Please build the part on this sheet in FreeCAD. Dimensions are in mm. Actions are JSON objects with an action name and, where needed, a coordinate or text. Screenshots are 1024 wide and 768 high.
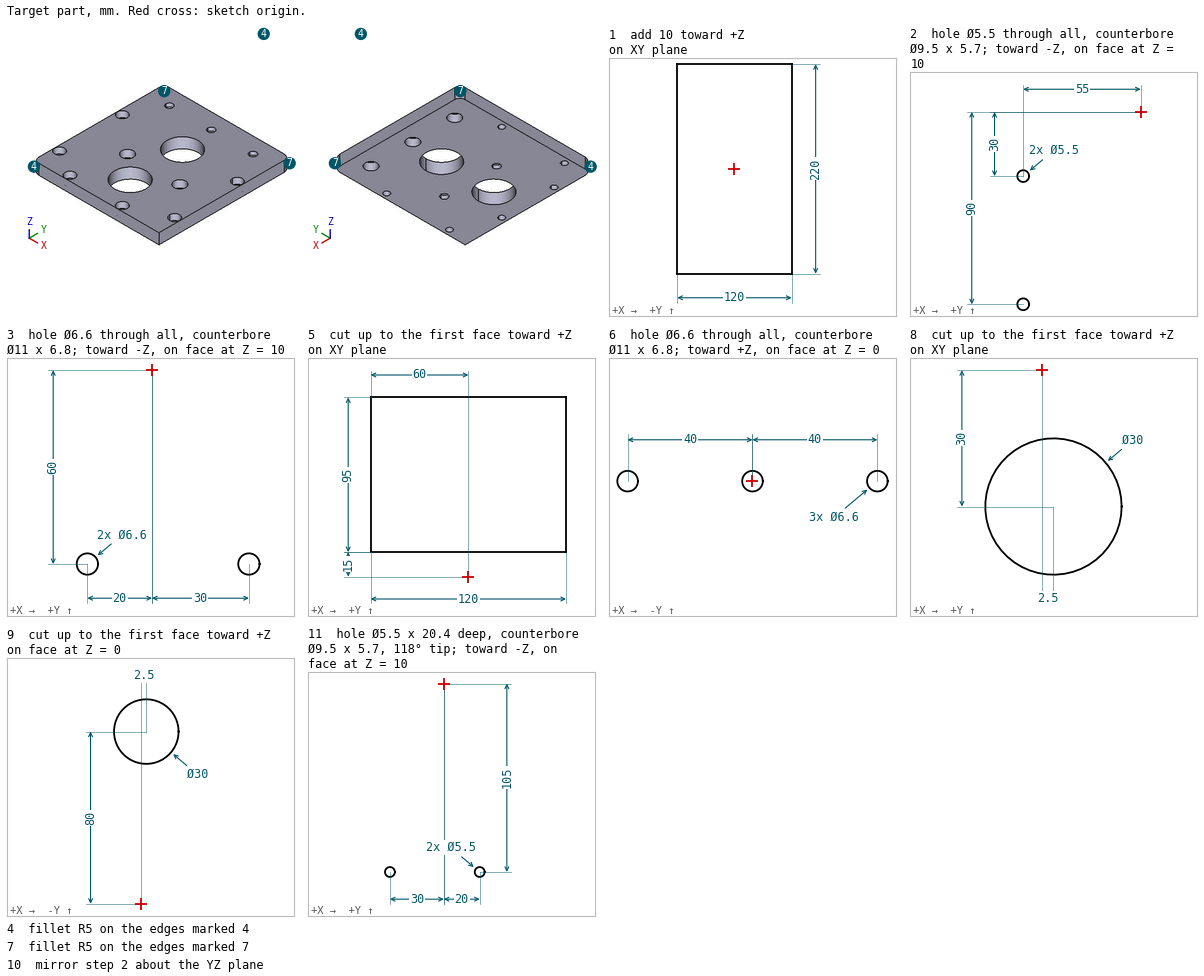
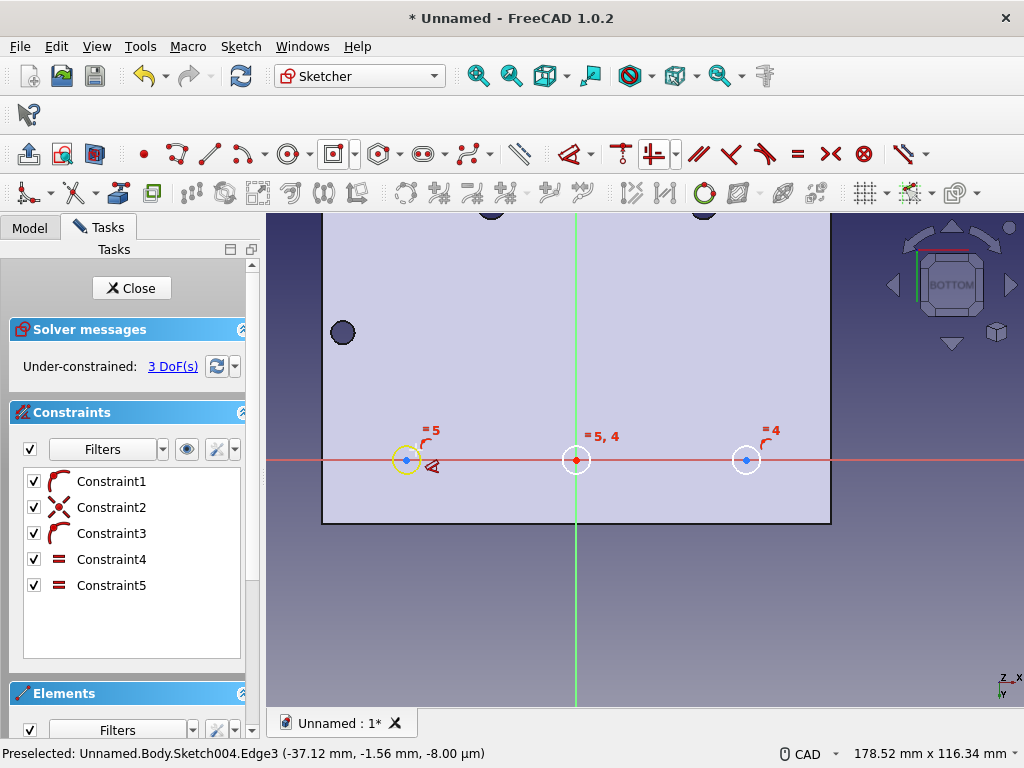
{"action": "scroll", "coordinate": [756, 450], "scroll_direction": "up", "scroll_amount": 2}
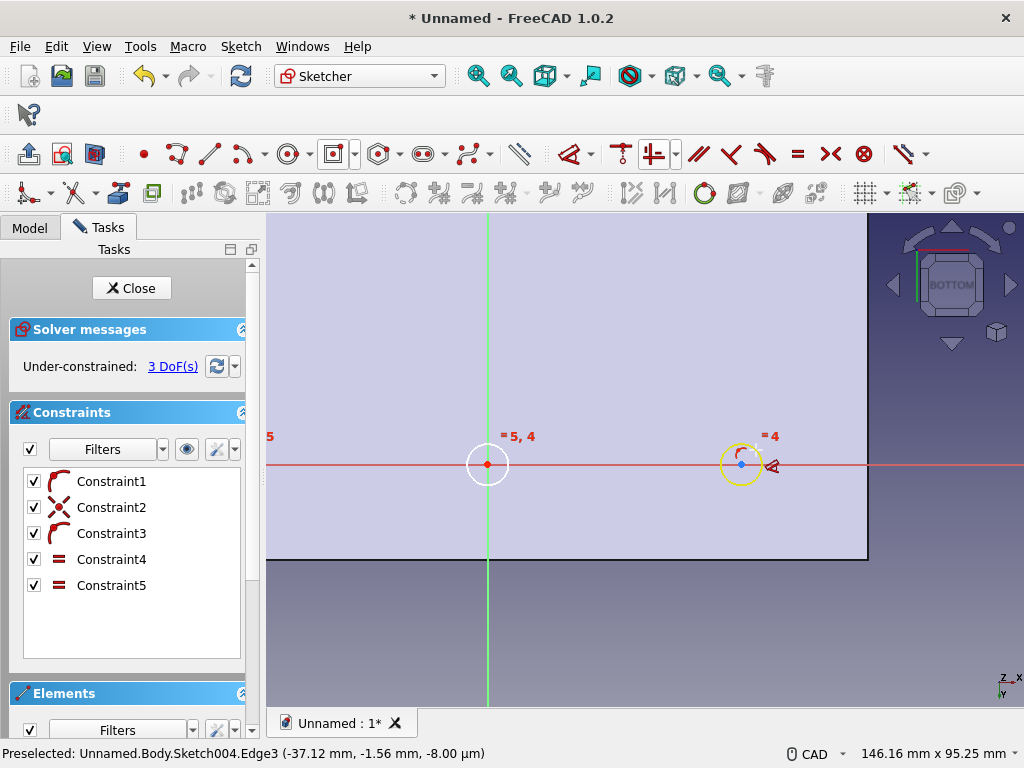
{"action": "left_click", "coordinate": [756, 450]}
{"action": "left_click", "coordinate": [779, 427]}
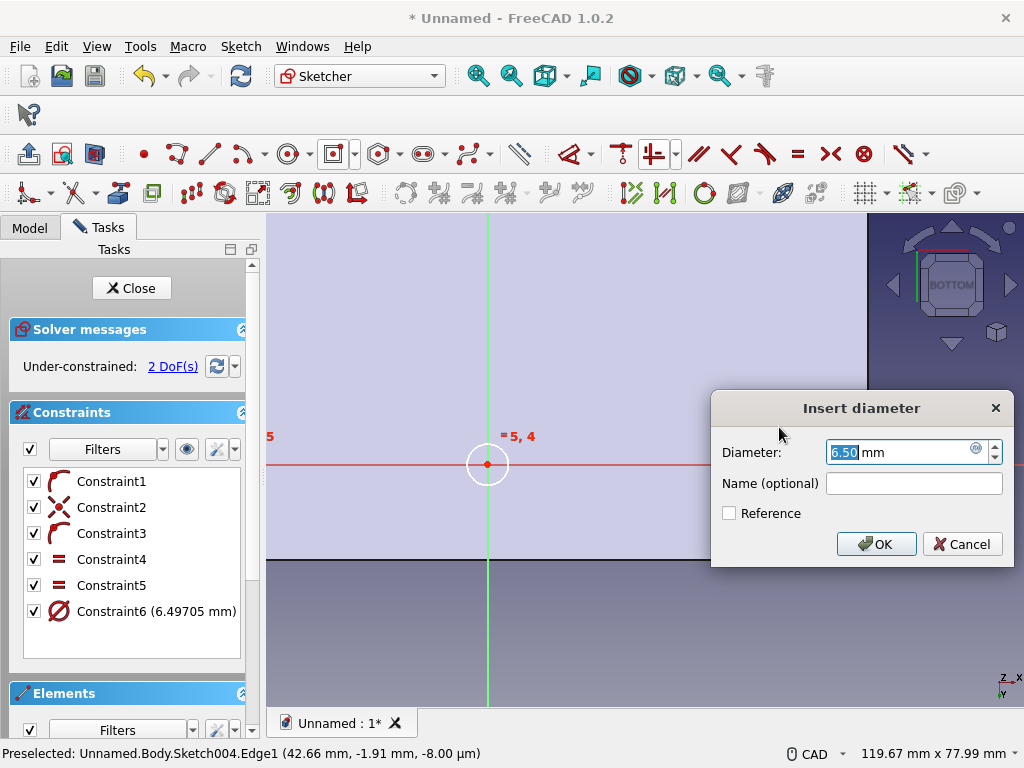
{"action": "type", "text": "6.6"}
{"action": "key", "text": "Return"}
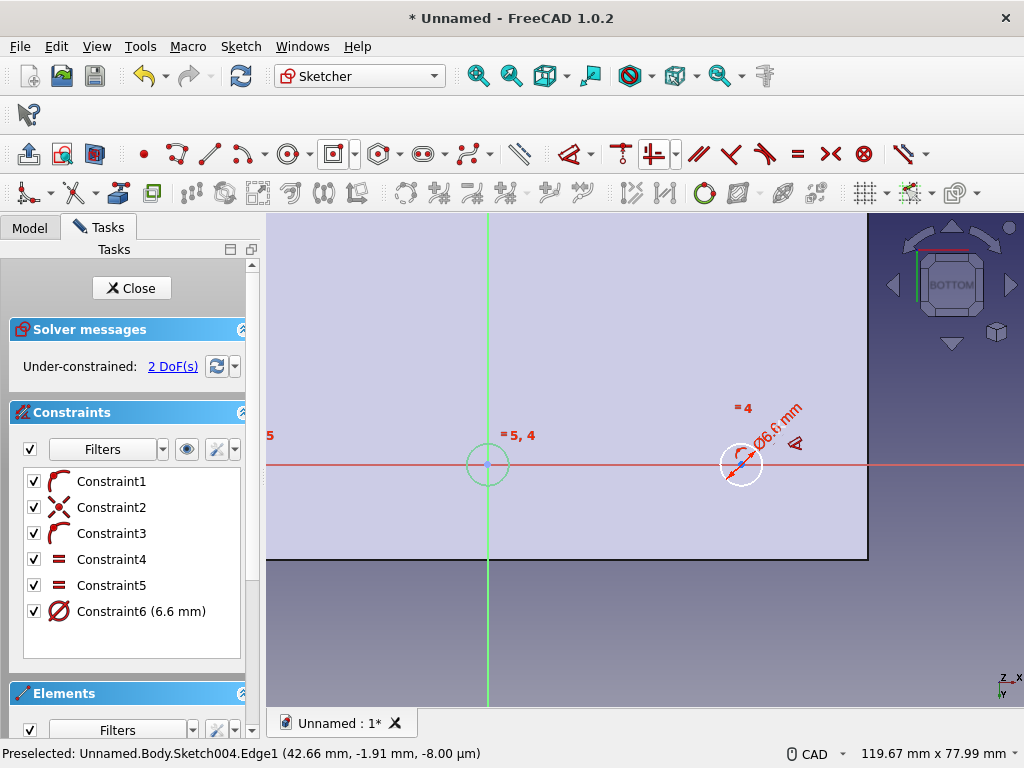
{"action": "left_click", "coordinate": [741, 465]}
{"action": "left_click", "coordinate": [615, 499]}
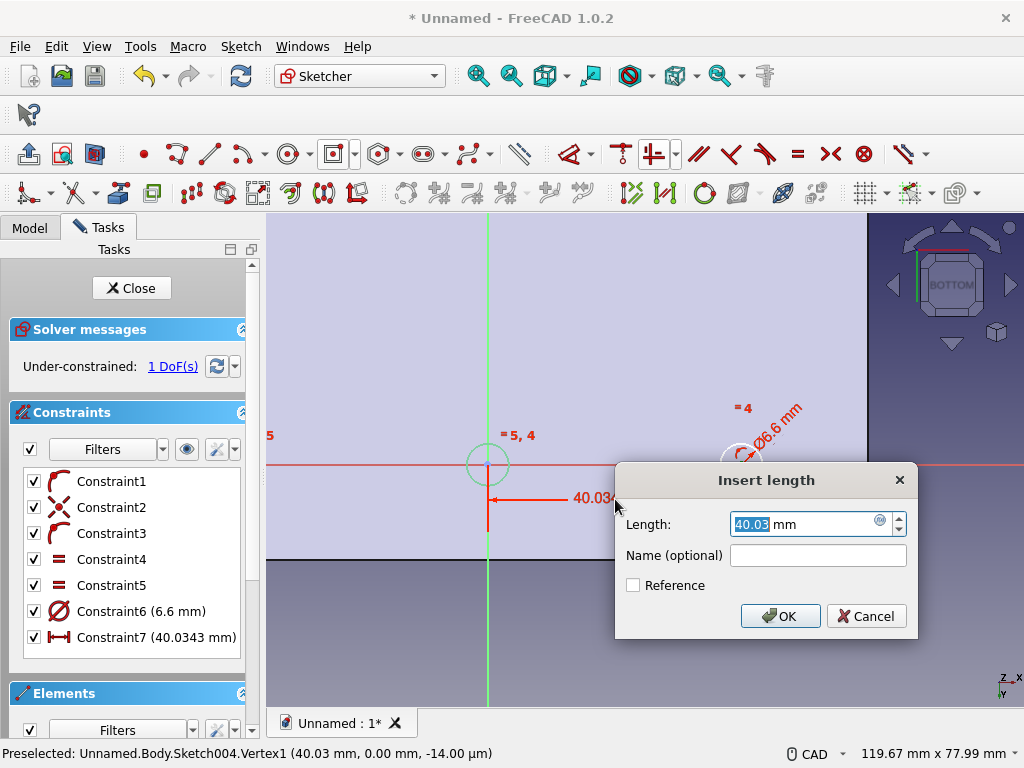
{"action": "type", "text": "40"}
{"action": "key", "text": "Return"}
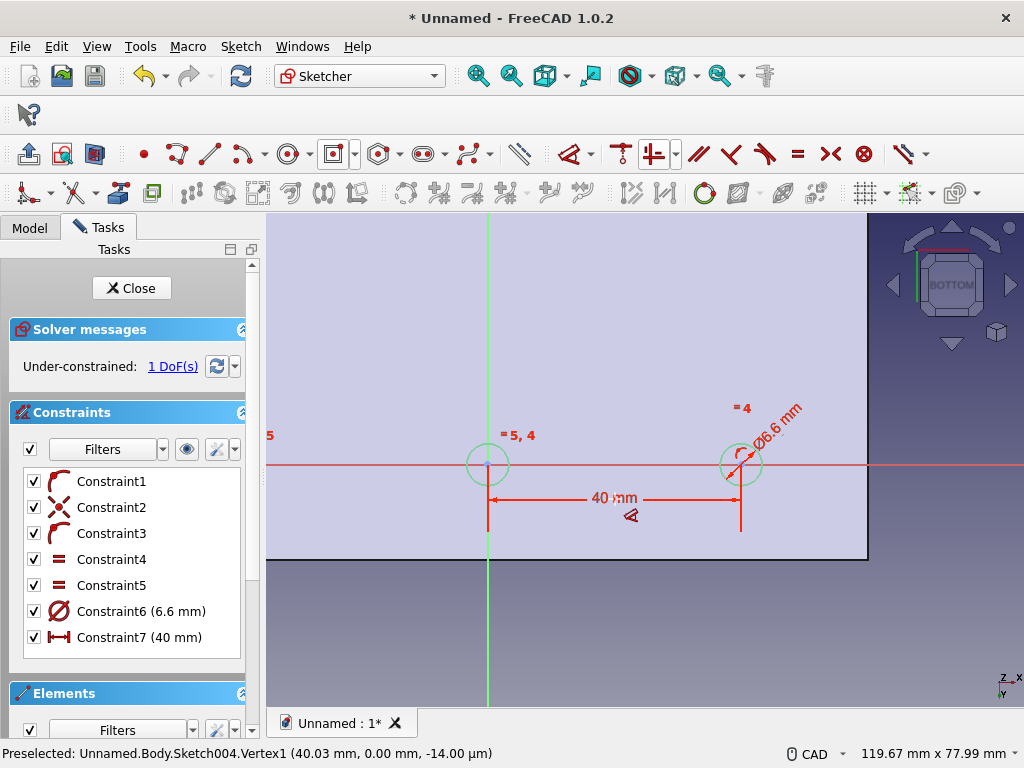
{"action": "scroll", "coordinate": [757, 450], "scroll_direction": "down", "scroll_amount": 2}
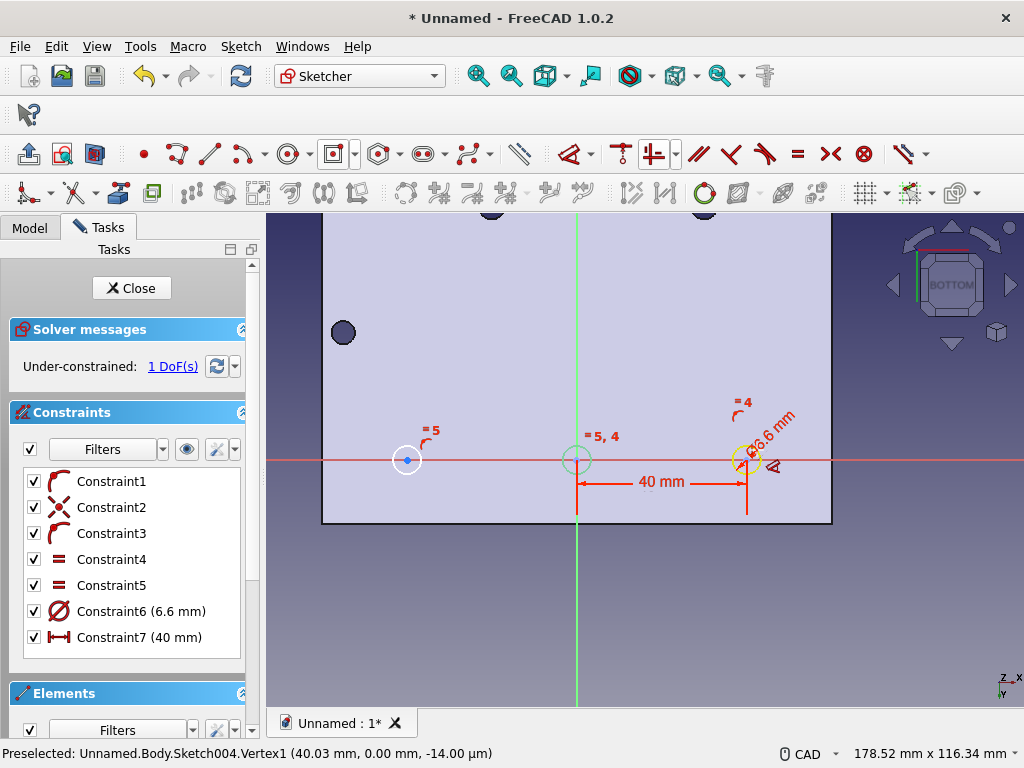
{"action": "left_click", "coordinate": [407, 460]}
{"action": "left_click", "coordinate": [492, 494]}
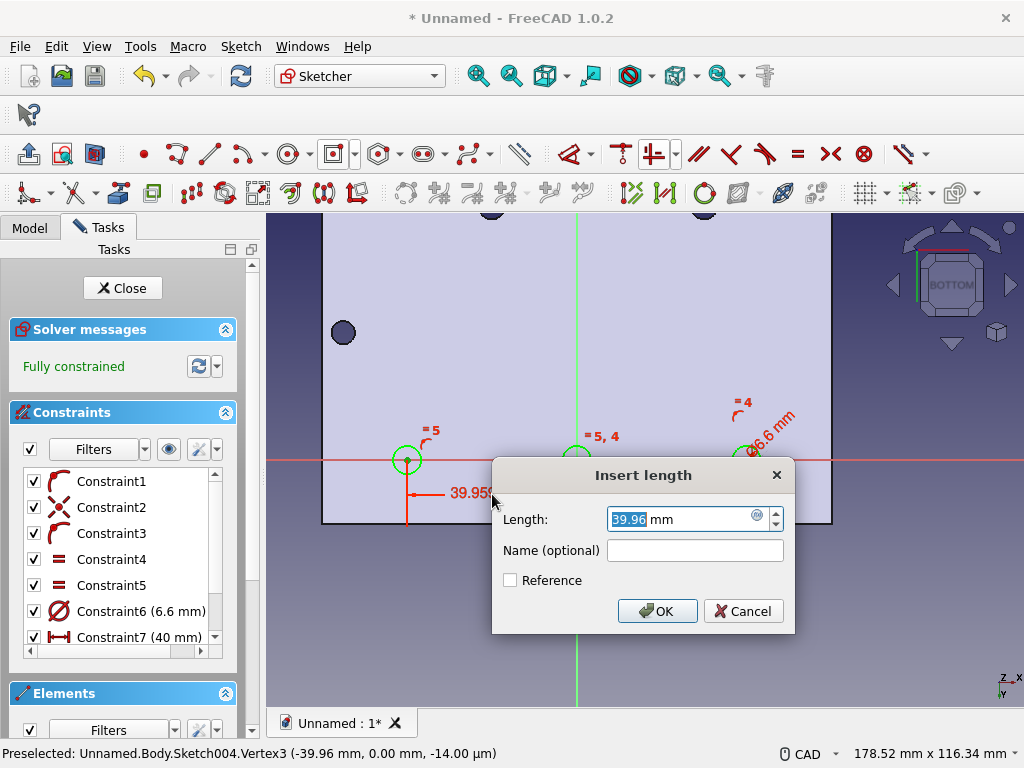
{"action": "type", "text": "40"}
{"action": "key", "text": "Return"}
{"action": "key", "text": "Escape"}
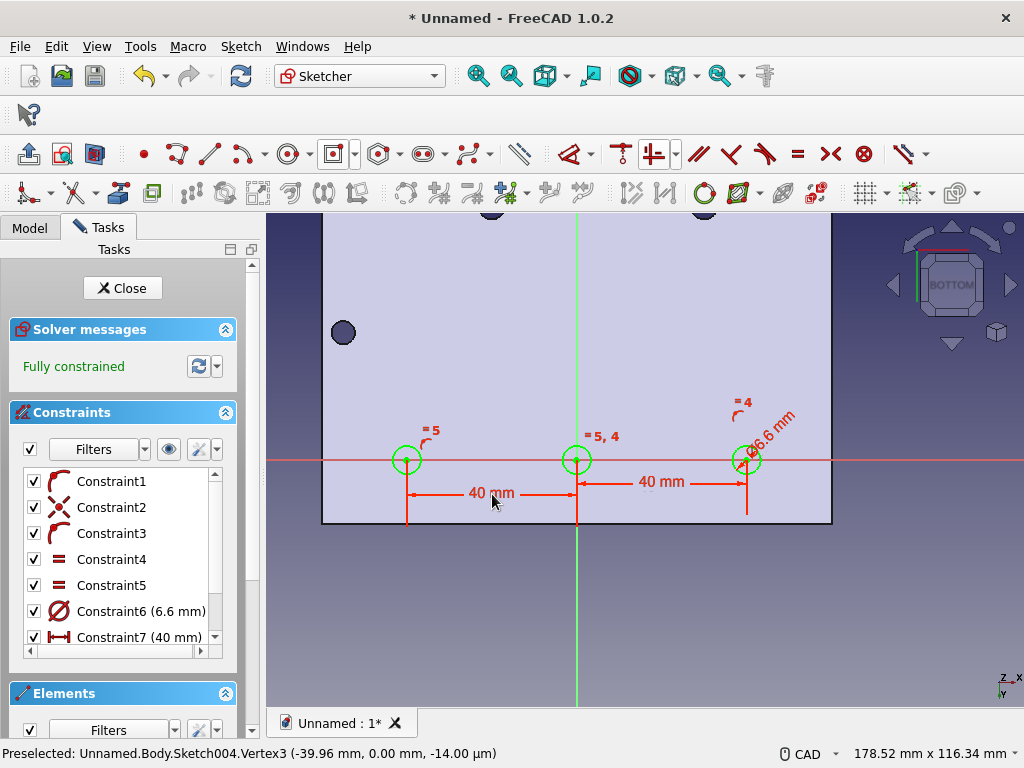
{"action": "left_click", "coordinate": [123, 288]}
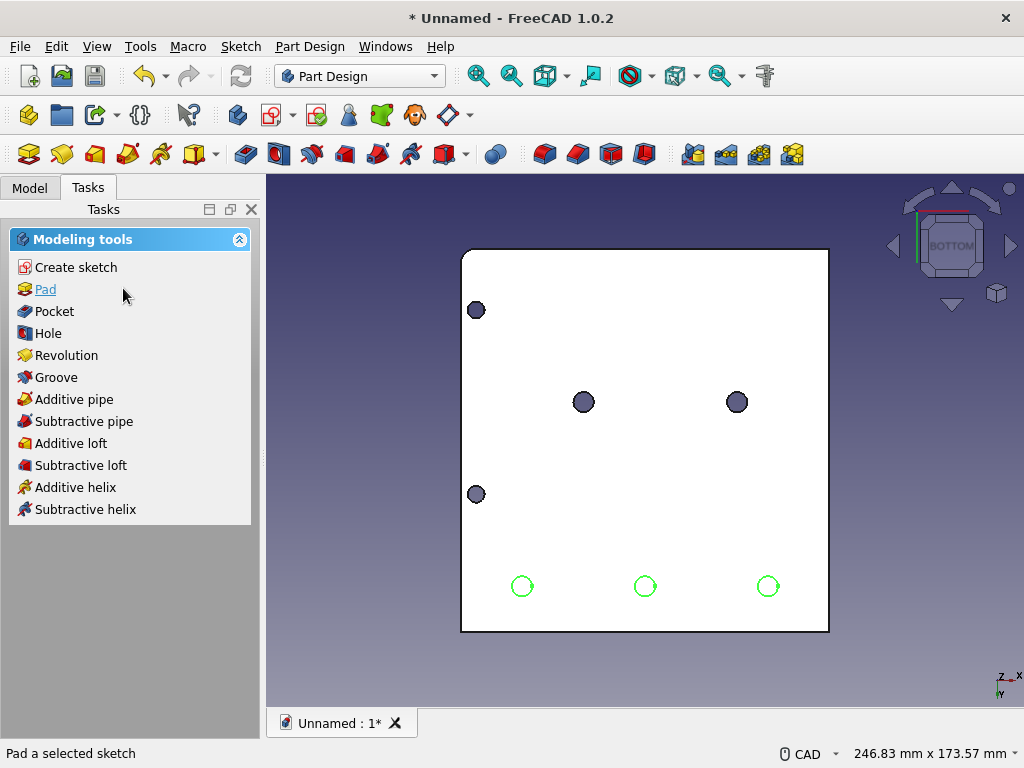
{"action": "left_click", "coordinate": [279, 154]}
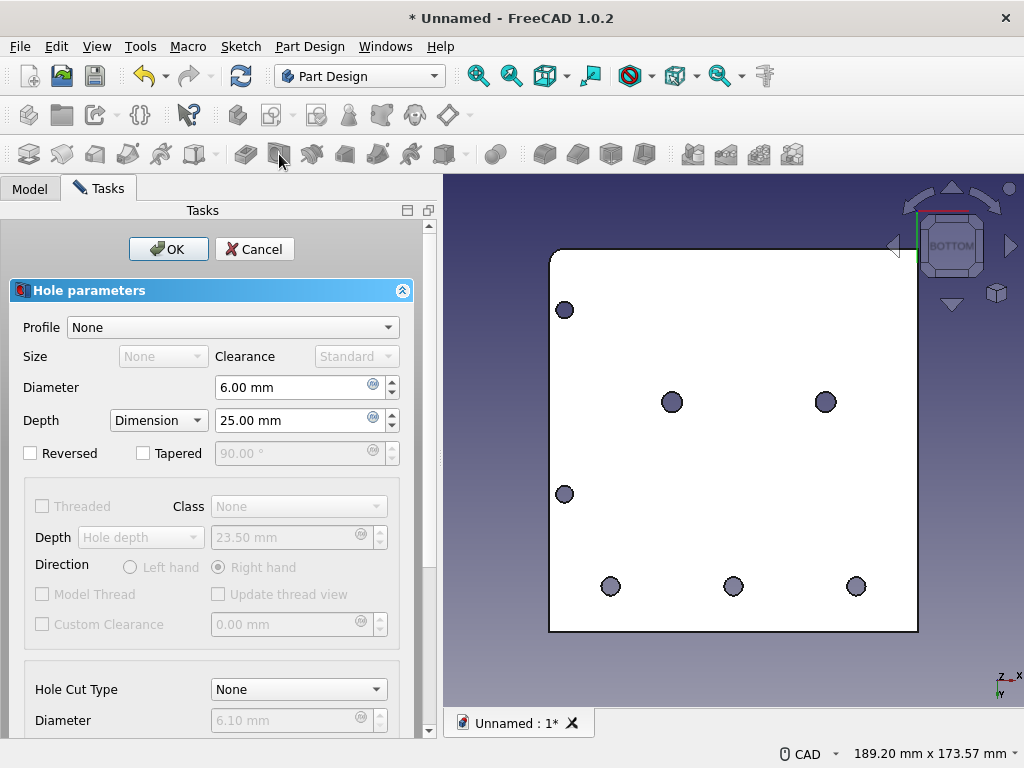
{"action": "triple_click", "coordinate": [300, 388]}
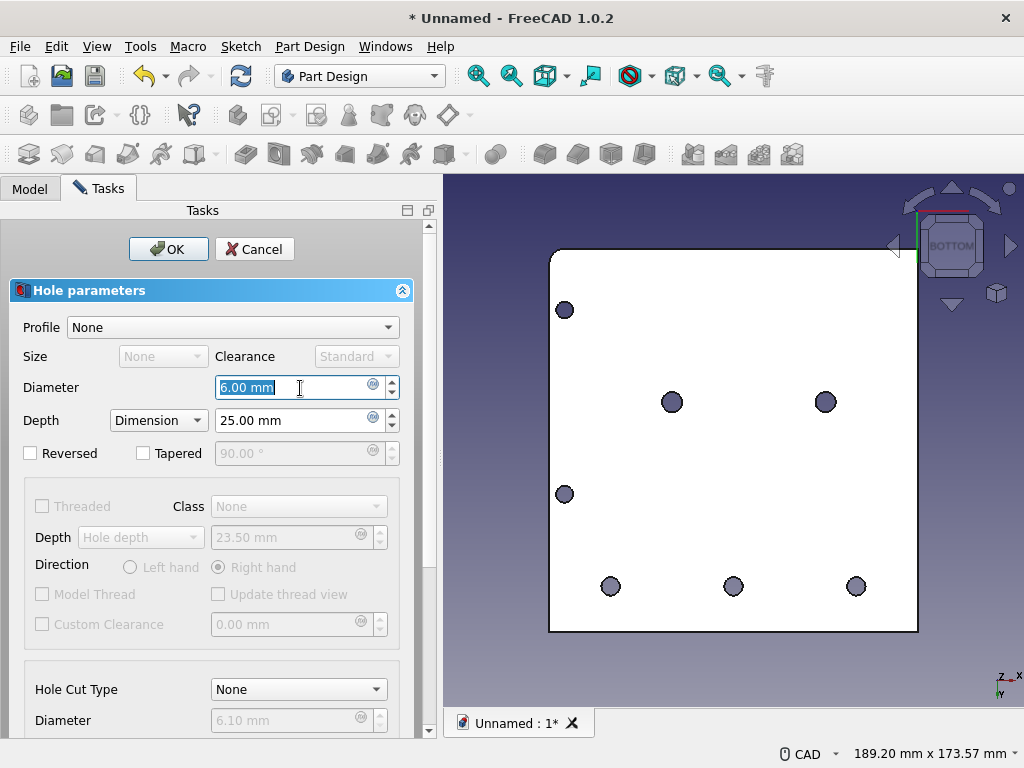
{"action": "type", "text": "6.6"}
{"action": "key", "text": "Tab"}